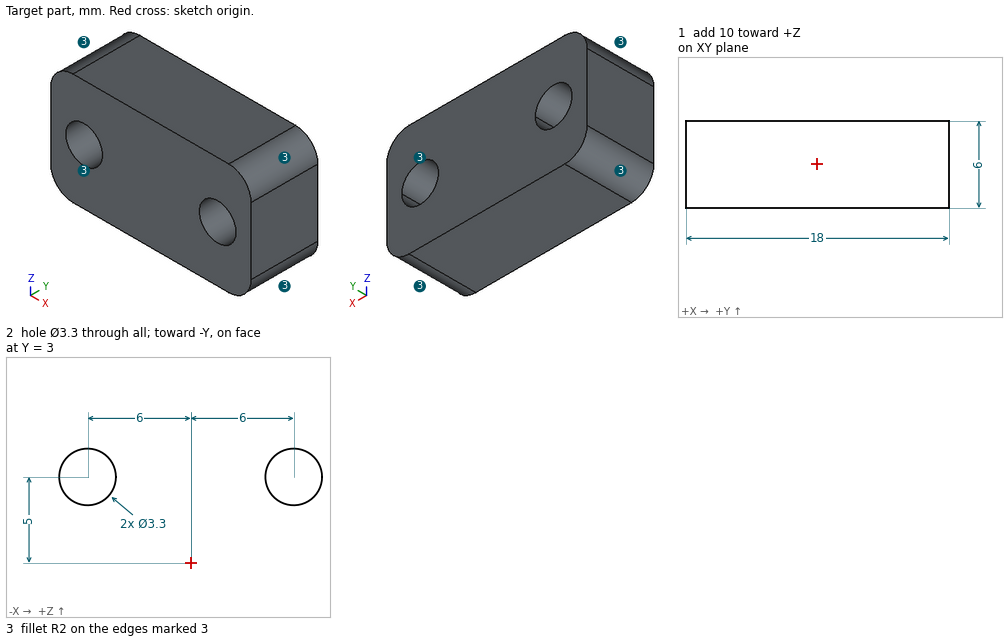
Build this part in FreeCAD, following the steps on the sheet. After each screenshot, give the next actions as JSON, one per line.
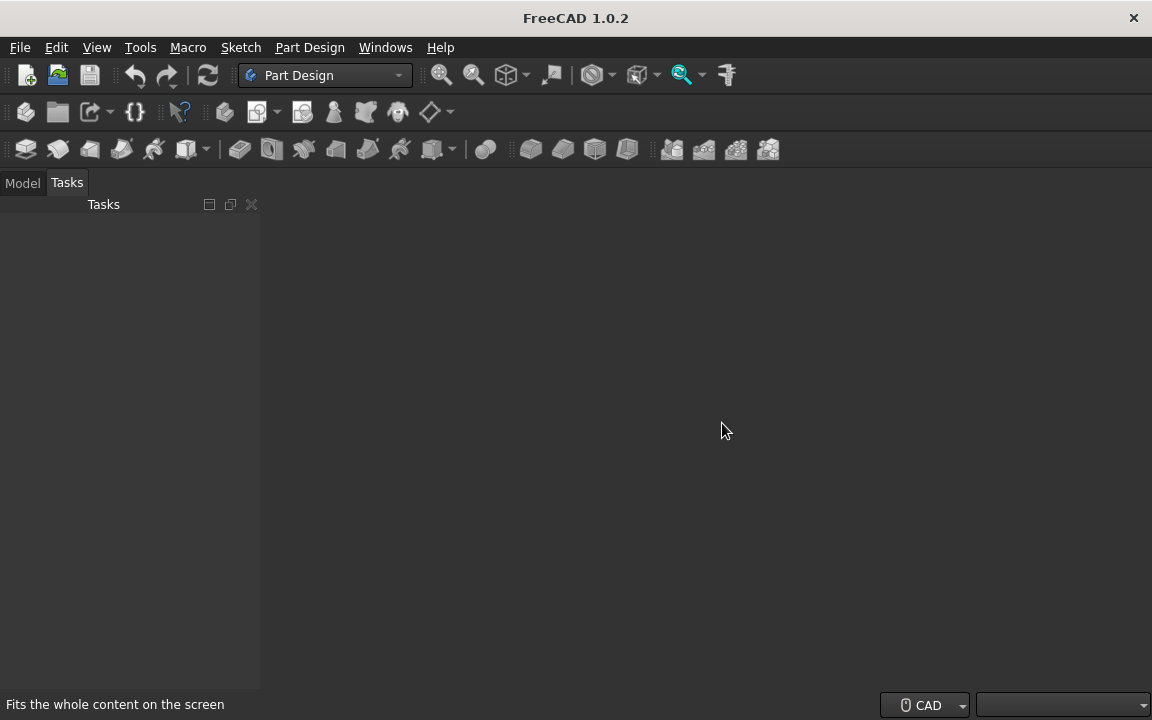
{"action": "left_click", "coordinate": [26, 76]}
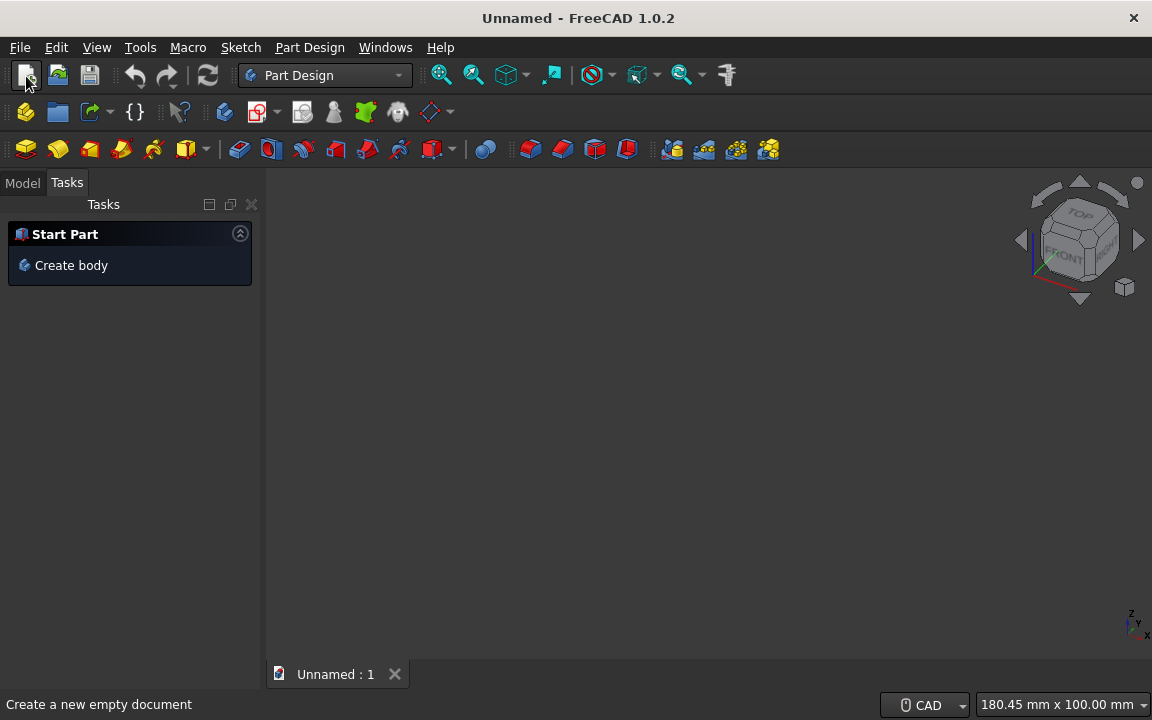
{"action": "left_click", "coordinate": [258, 112]}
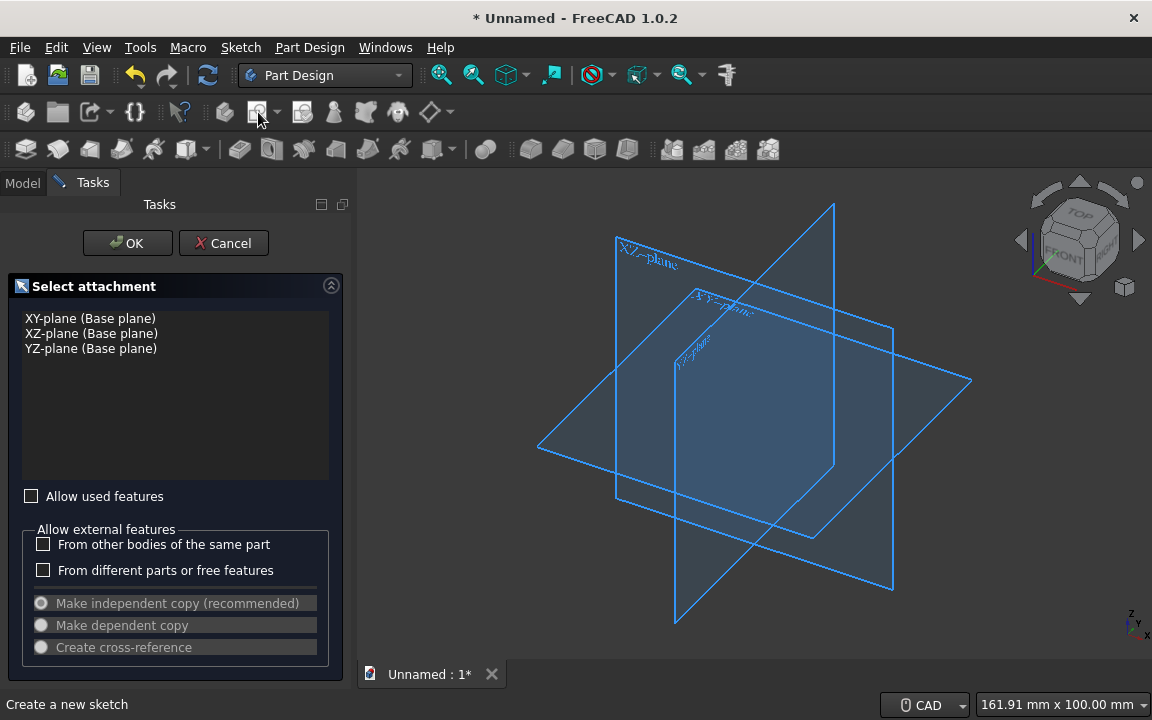
{"action": "left_click", "coordinate": [82, 318]}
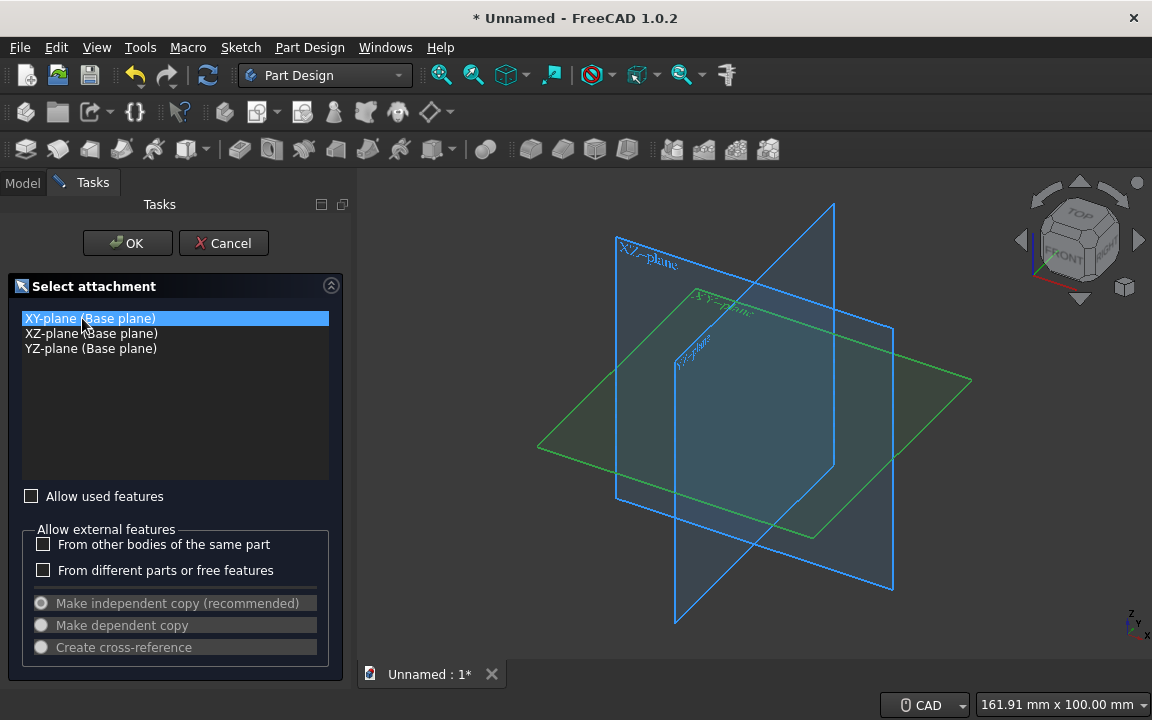
{"action": "left_click", "coordinate": [128, 243]}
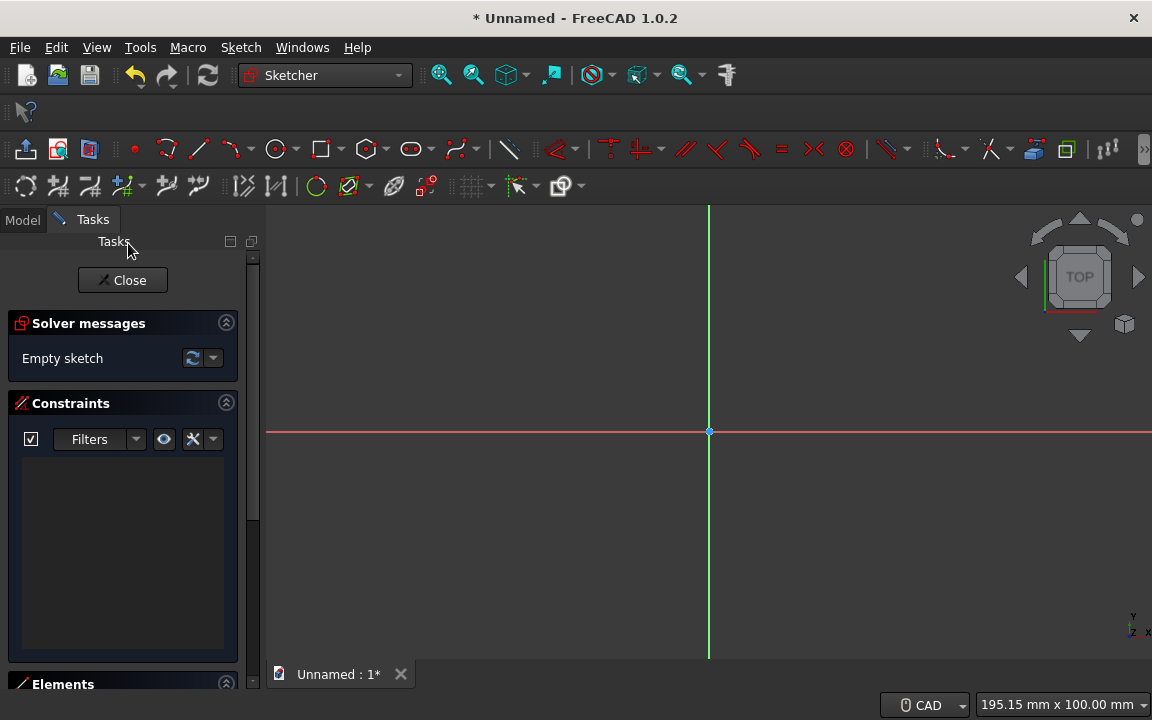
{"action": "scroll", "coordinate": [723, 432], "scroll_direction": "up", "scroll_amount": 9}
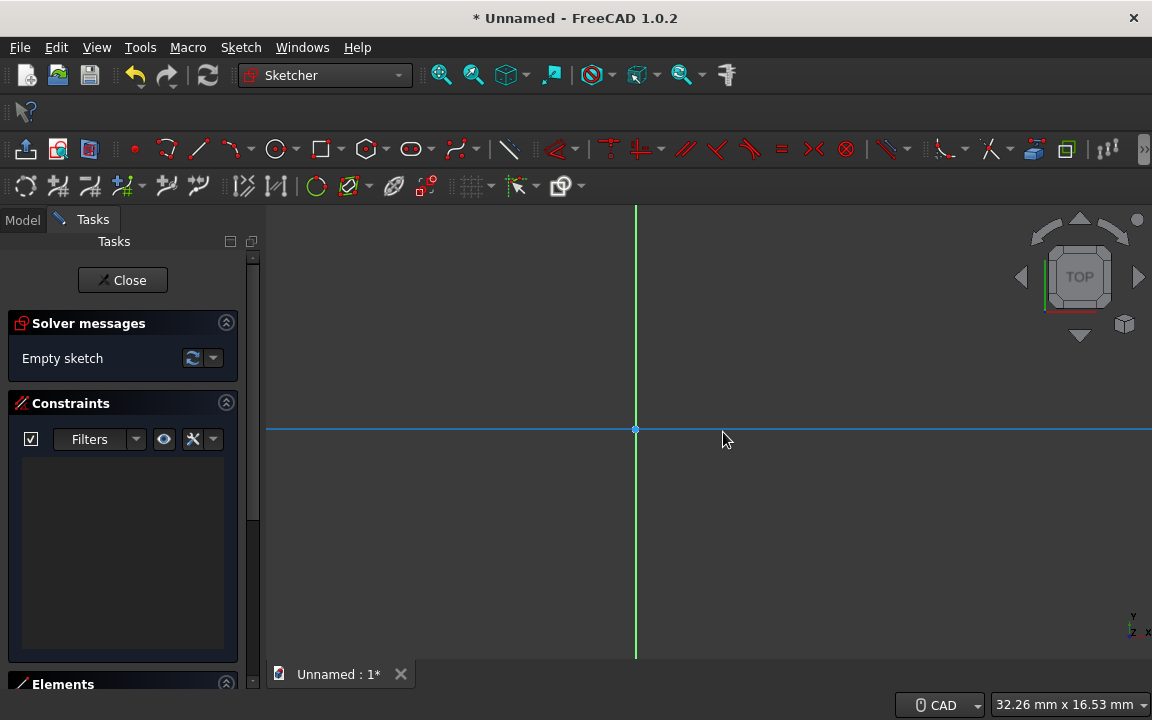
{"action": "key", "text": "g v"}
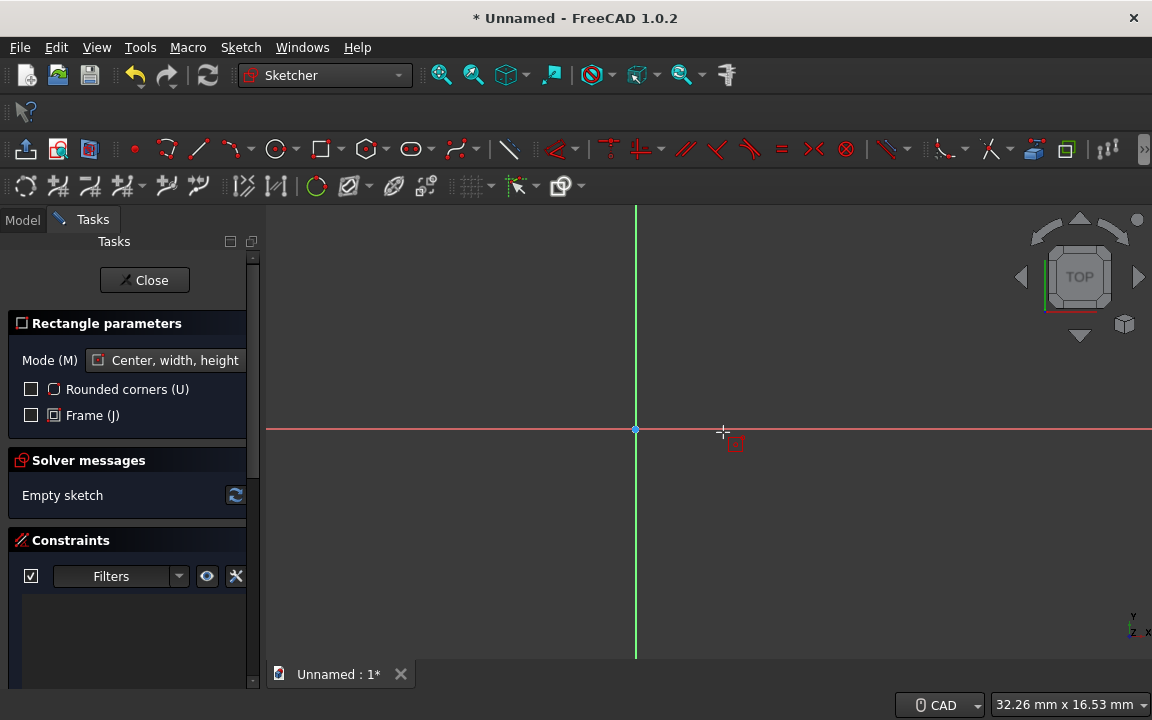
{"action": "left_click", "coordinate": [636, 429]}
{"action": "mouse_move", "coordinate": [883, 347]}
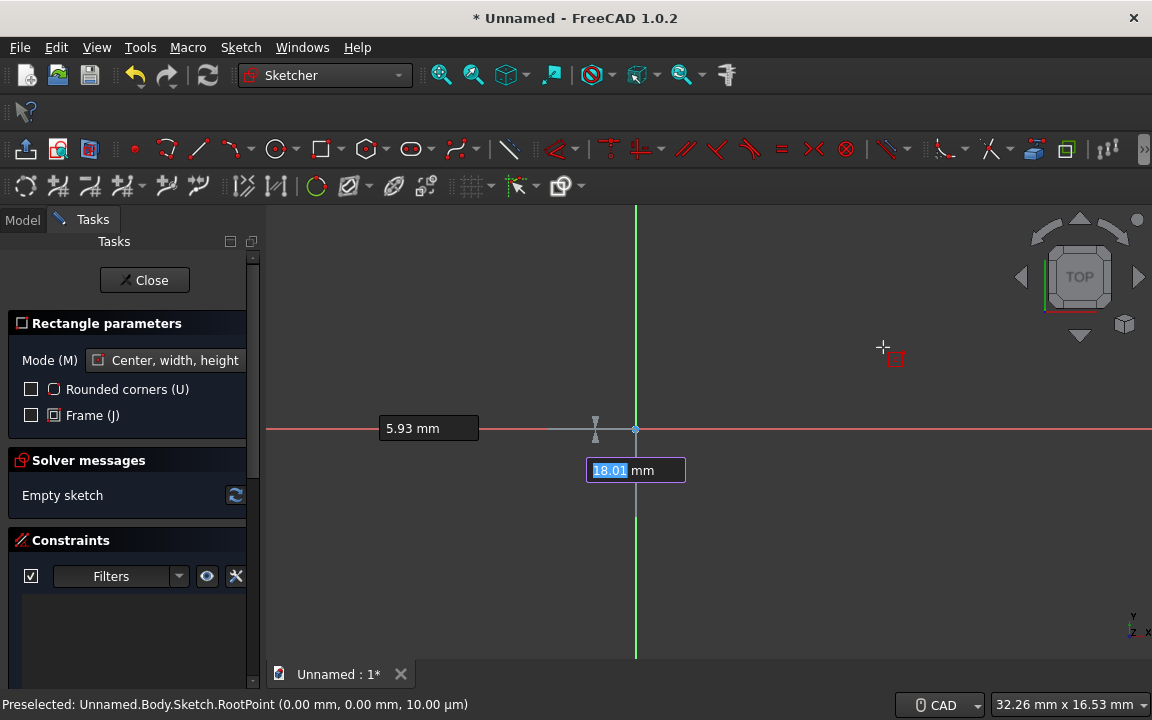
{"action": "type", "text": "18"}
{"action": "key", "text": "Tab"}
{"action": "type", "text": "6"}
{"action": "key", "text": "Return"}
{"action": "key", "text": "Escape"}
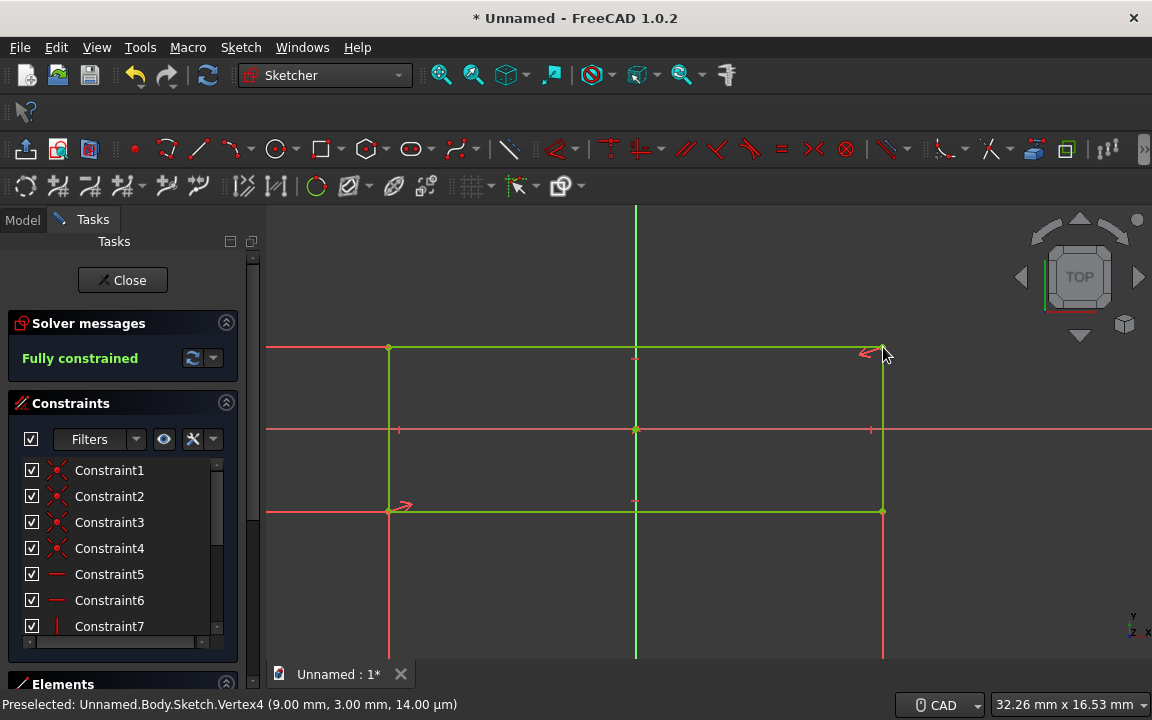
{"action": "left_click", "coordinate": [123, 280]}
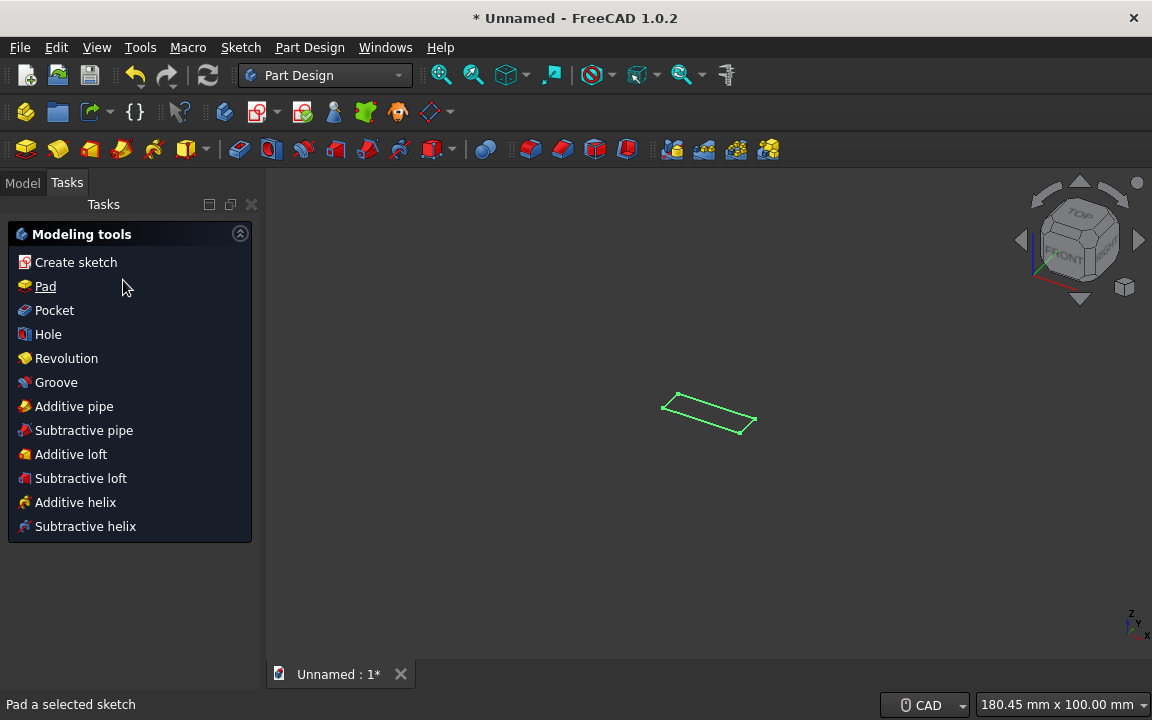
{"action": "left_click", "coordinate": [26, 150]}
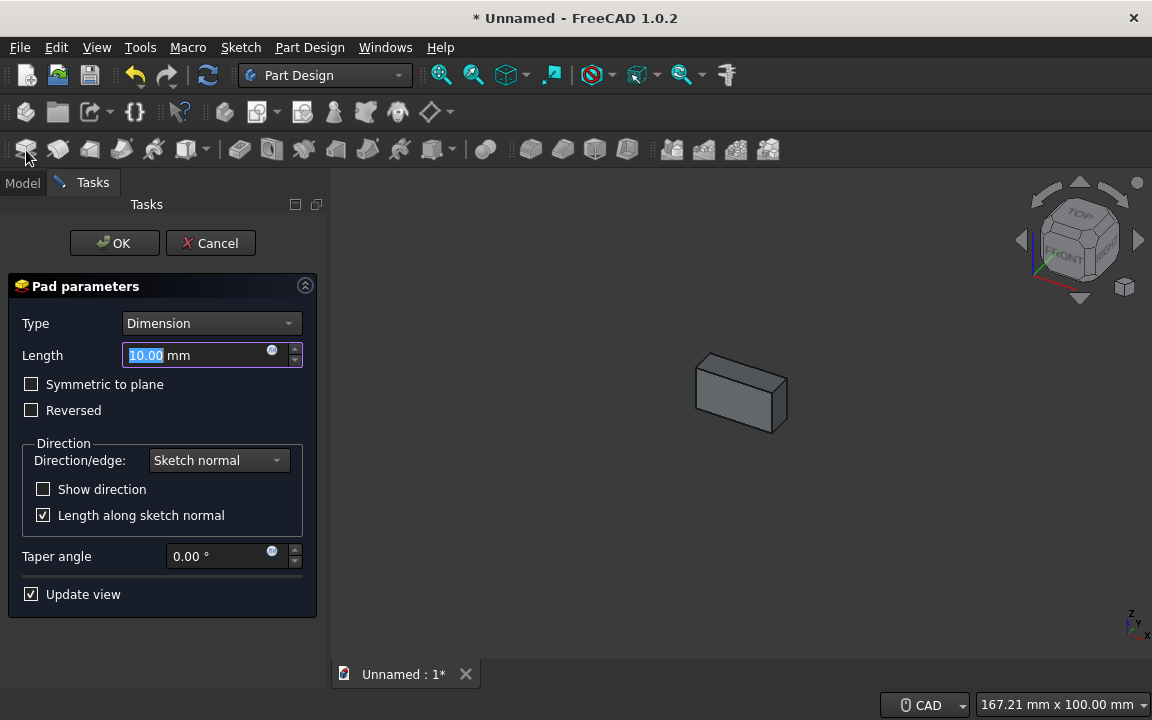
{"action": "type", "text": "10"}
{"action": "key", "text": "Tab"}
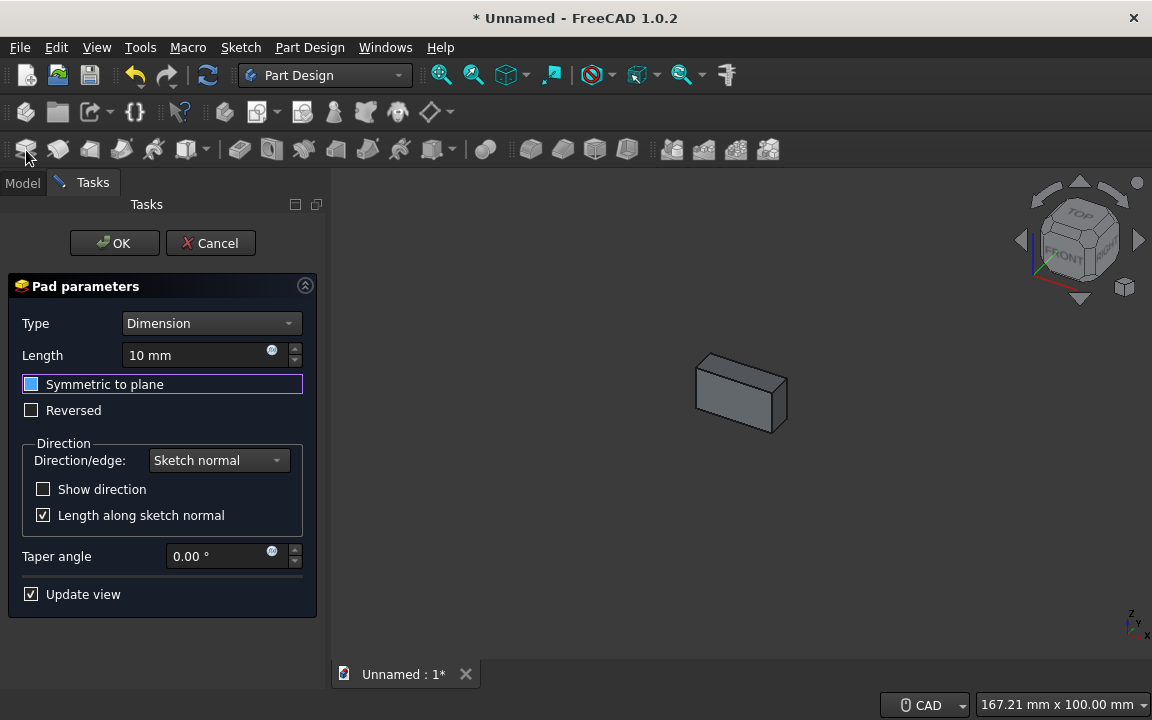
{"action": "left_click", "coordinate": [115, 243]}